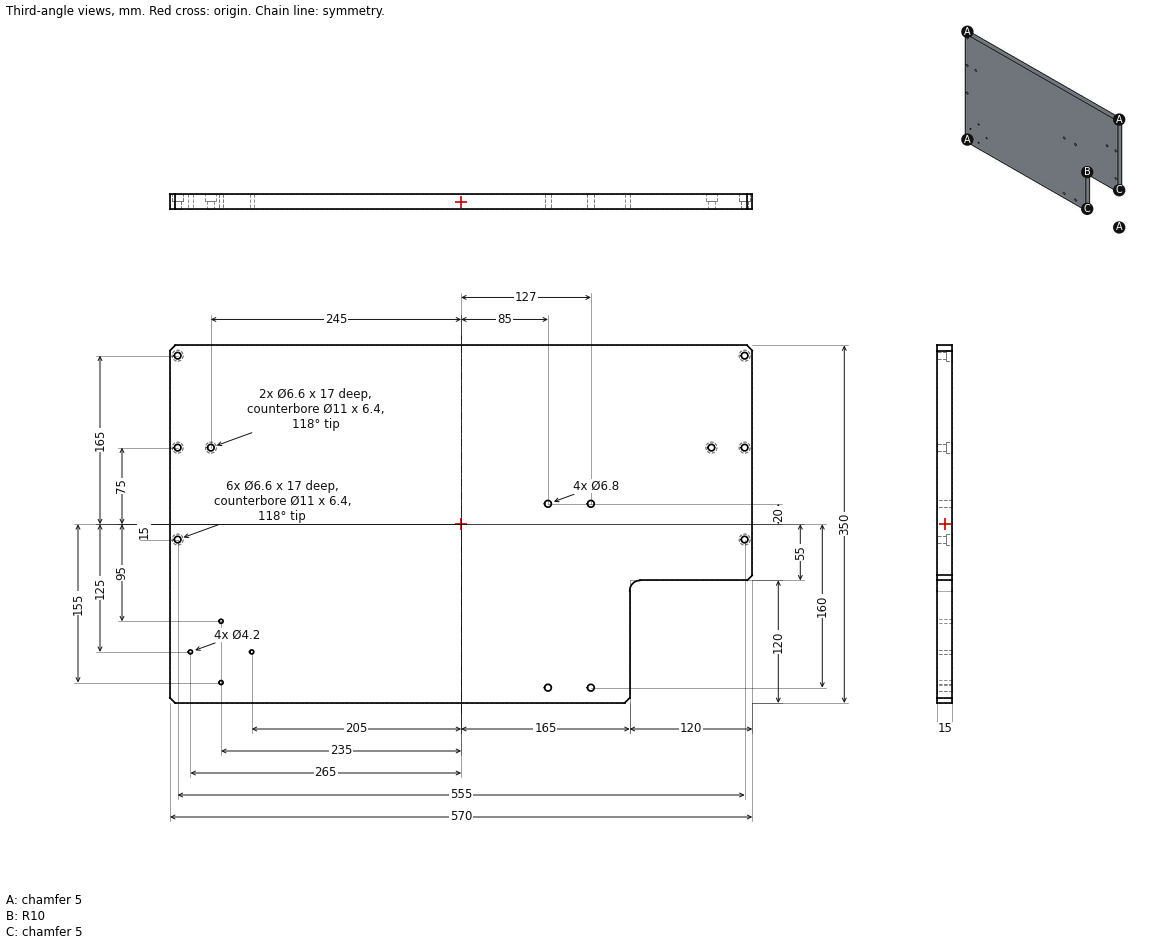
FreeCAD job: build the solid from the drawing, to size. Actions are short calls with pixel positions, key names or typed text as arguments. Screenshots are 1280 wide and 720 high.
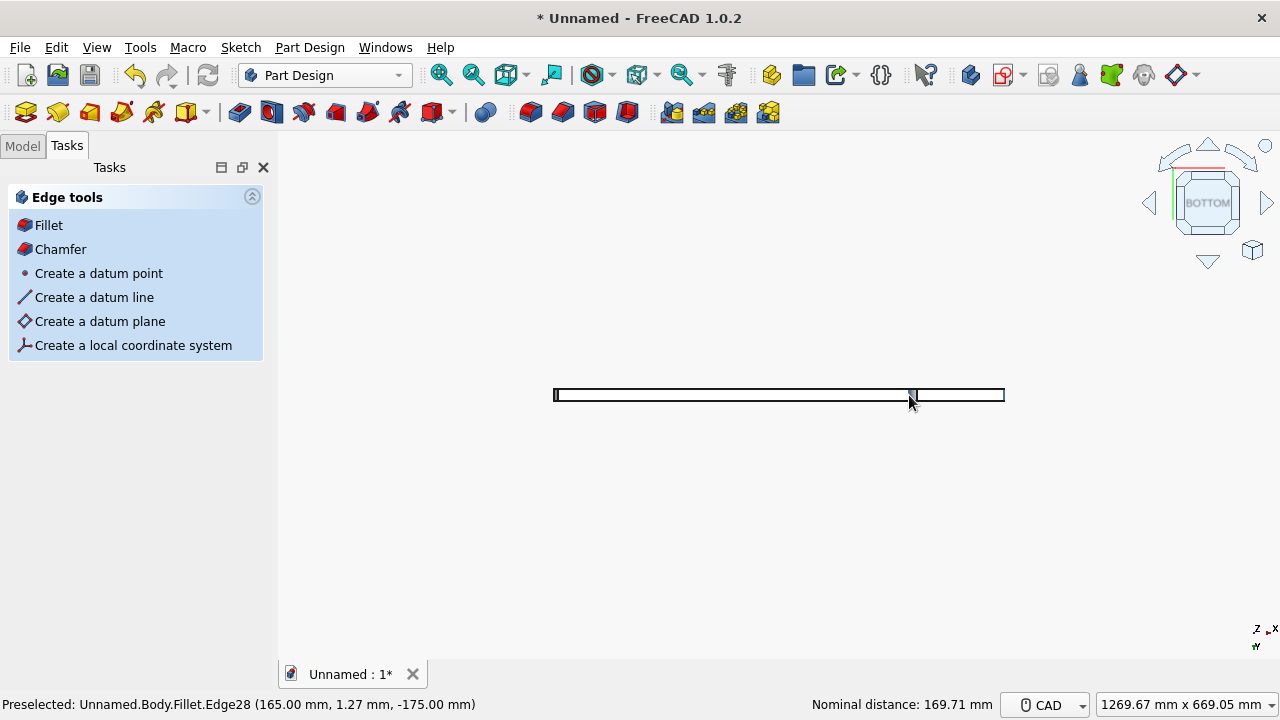
click(564, 112)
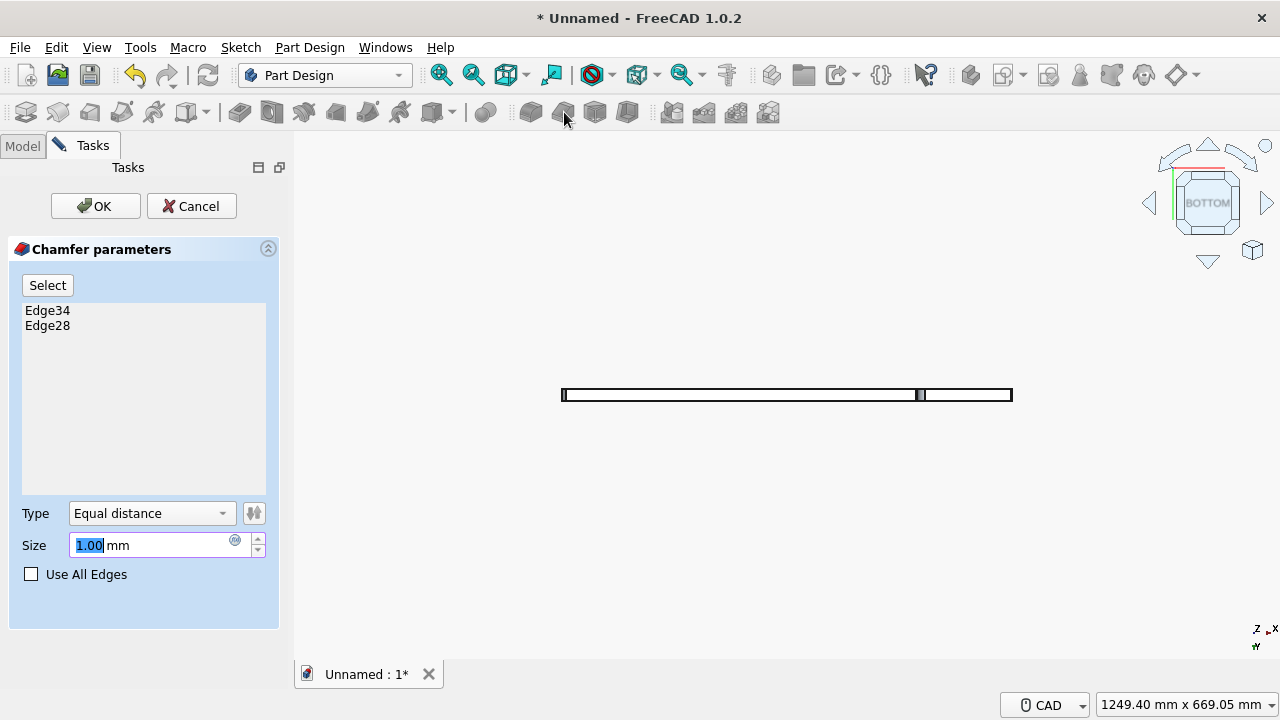
text(5)
key(Tab)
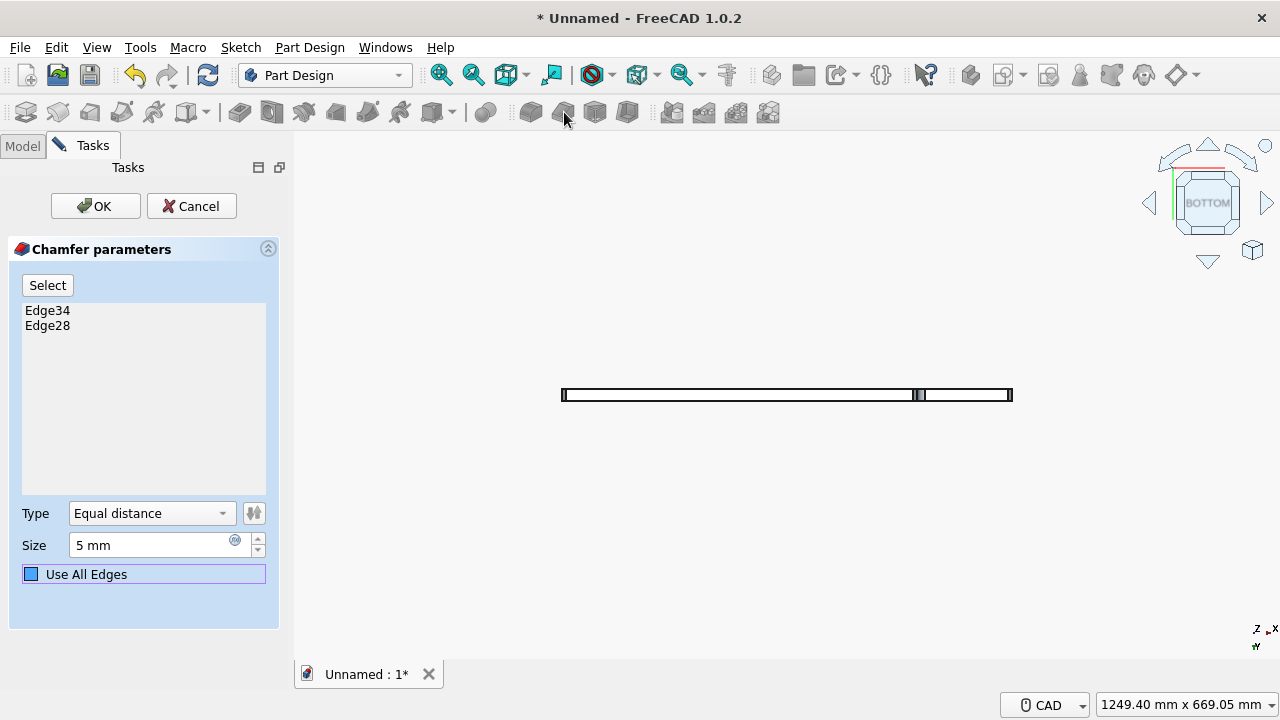
click(96, 206)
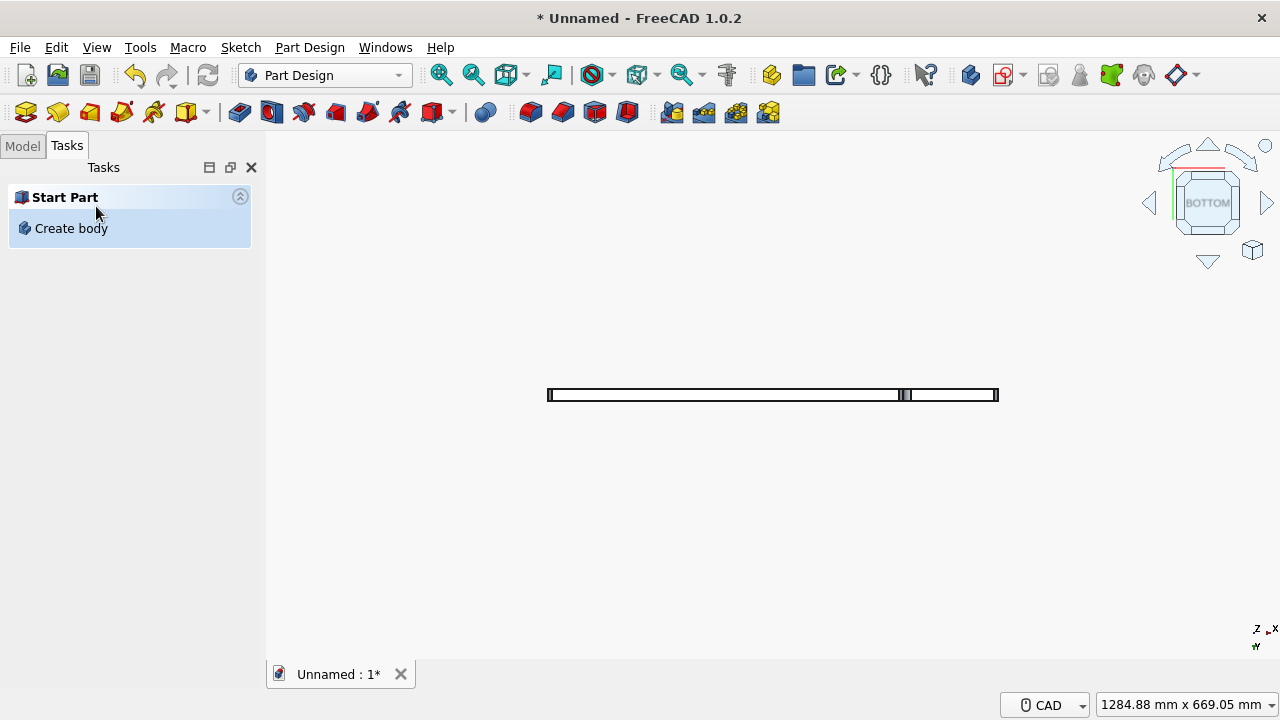
key(0)